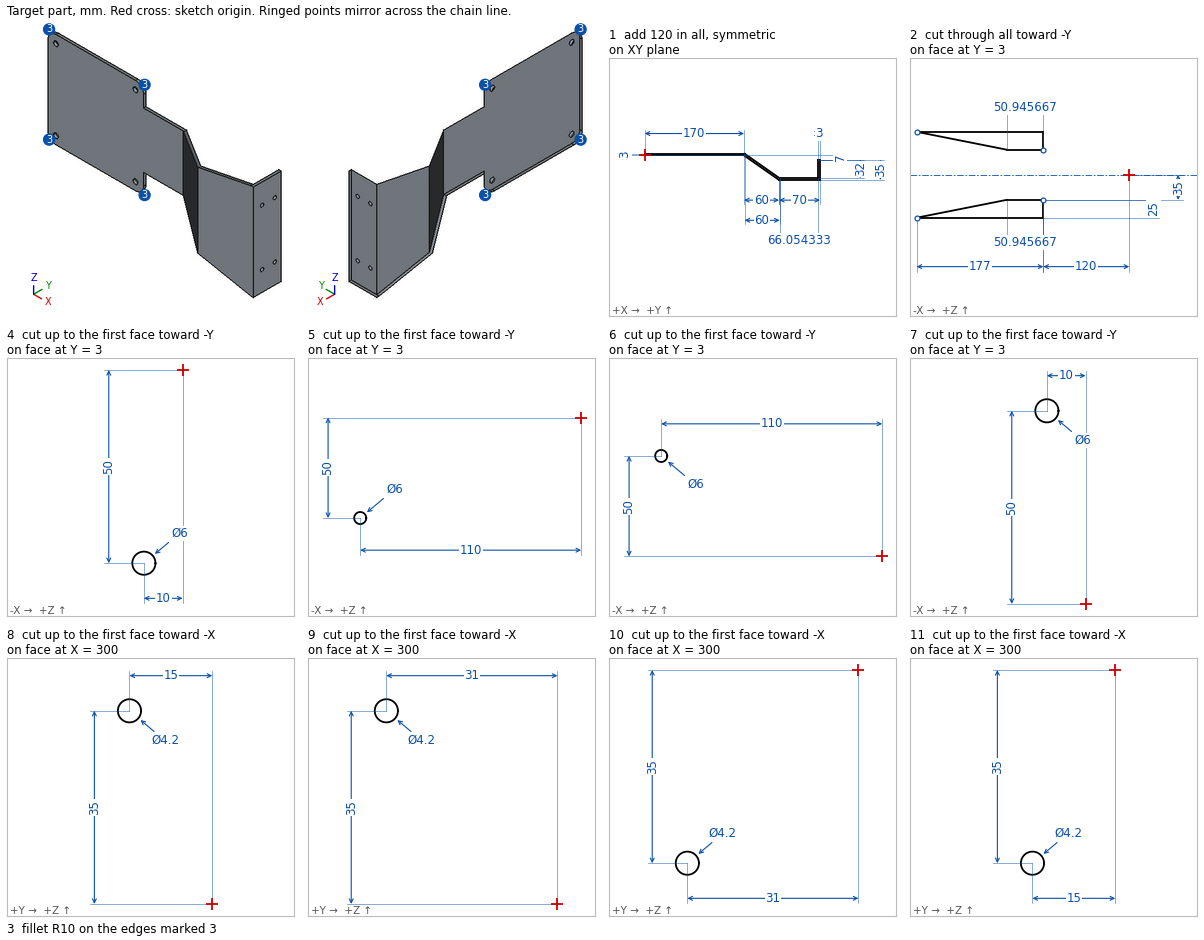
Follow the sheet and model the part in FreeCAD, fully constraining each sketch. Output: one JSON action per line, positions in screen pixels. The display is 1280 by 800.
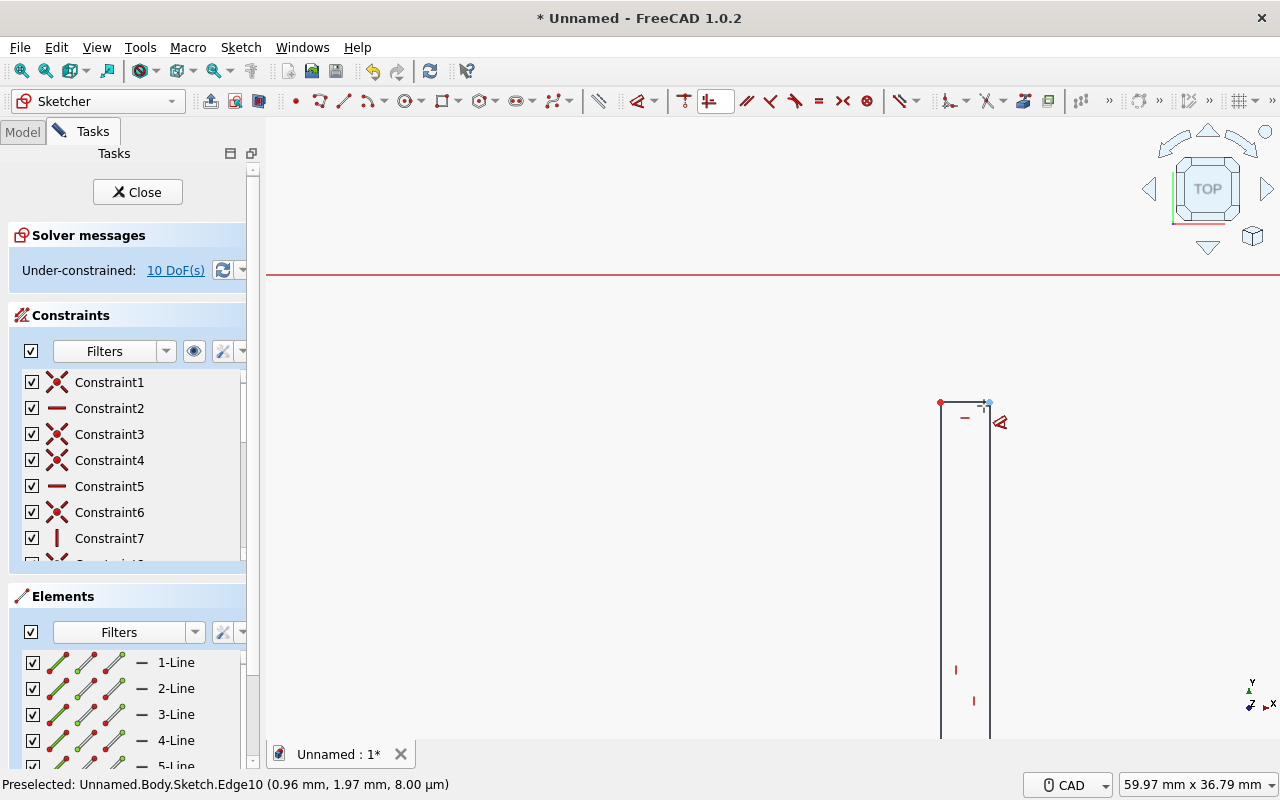
{"action": "left_click", "coordinate": [975, 402]}
{"action": "left_click", "coordinate": [965, 368]}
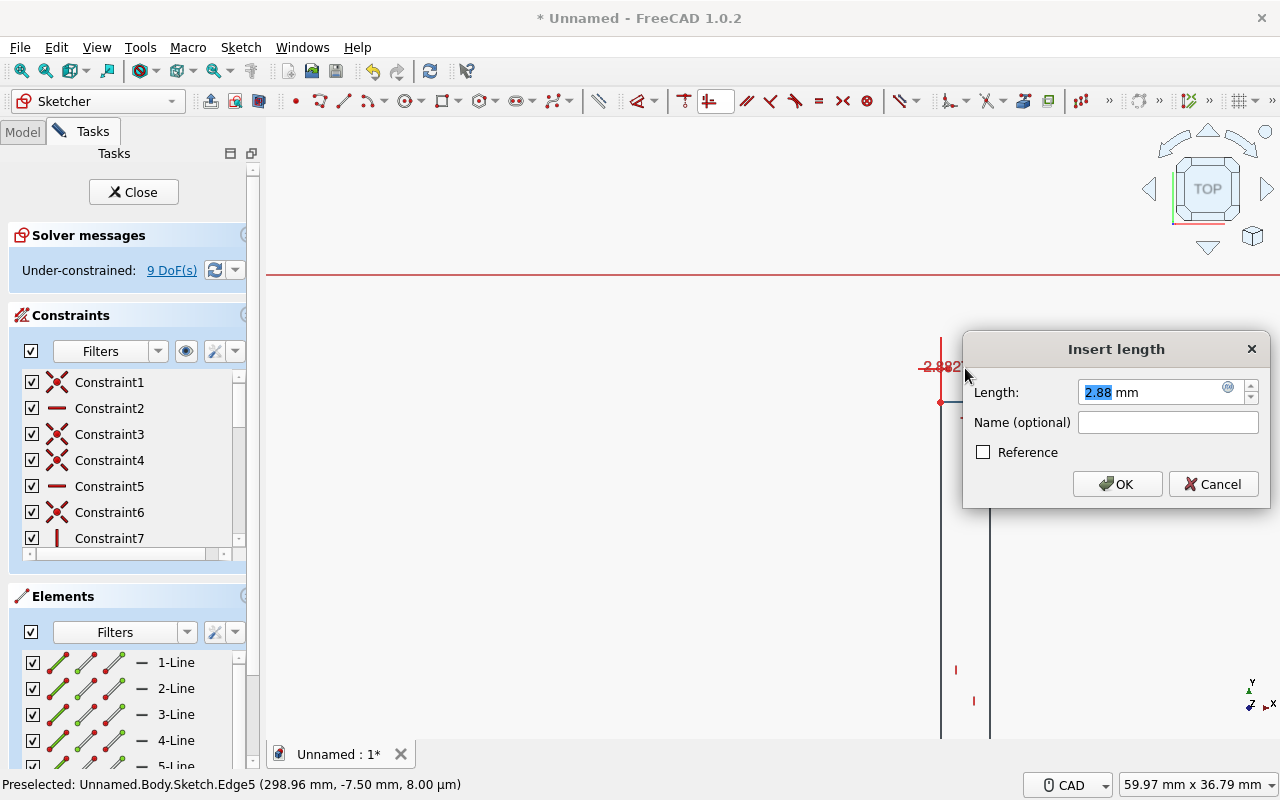
{"action": "type", "text": "3"}
{"action": "key", "text": "Return"}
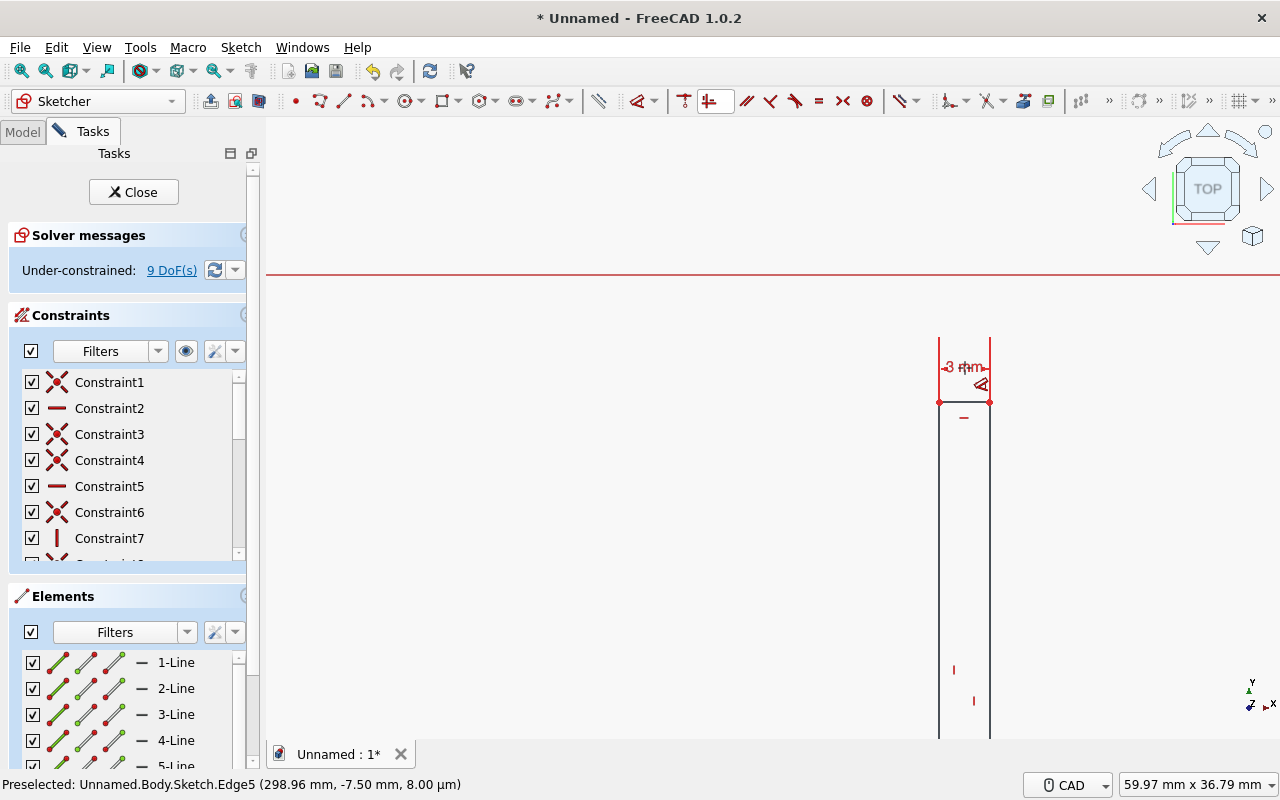
{"action": "scroll", "coordinate": [985, 406], "scroll_direction": "down", "scroll_amount": 11}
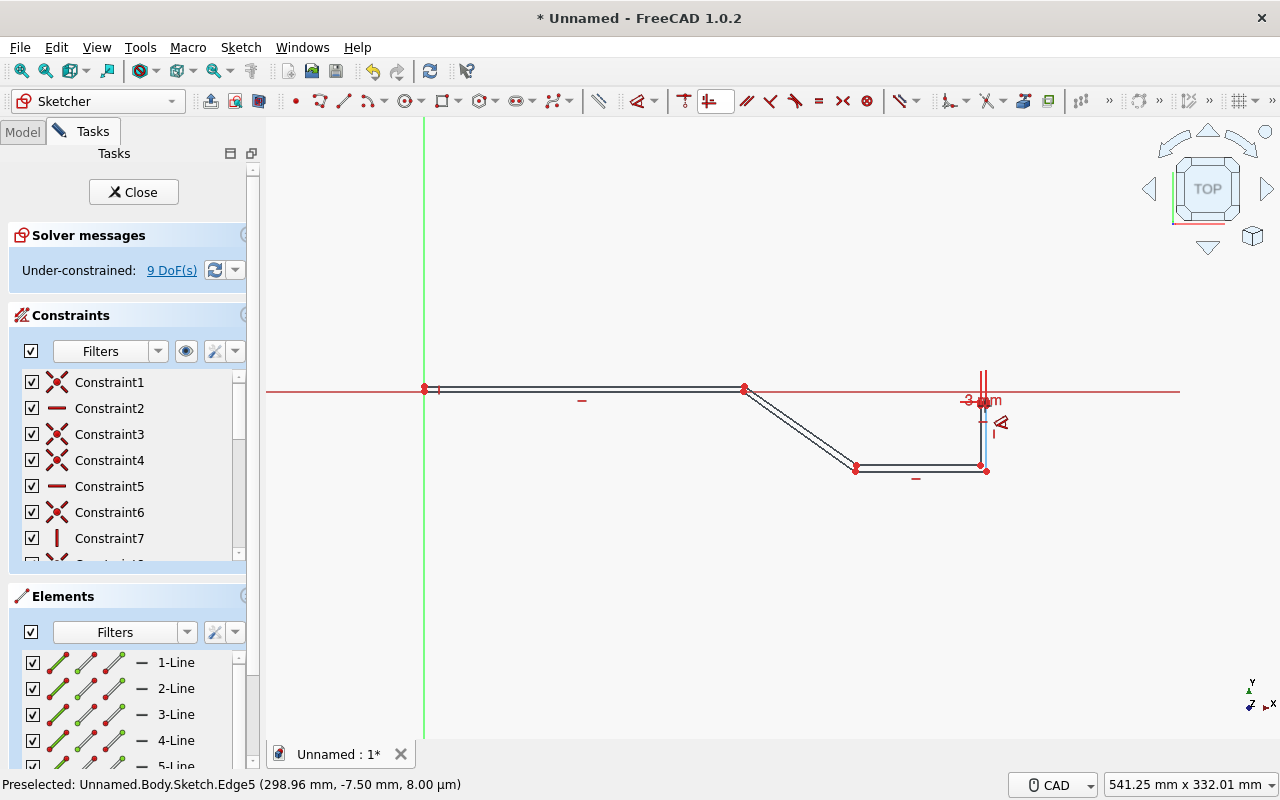
{"action": "scroll", "coordinate": [424, 388], "scroll_direction": "up", "scroll_amount": 11}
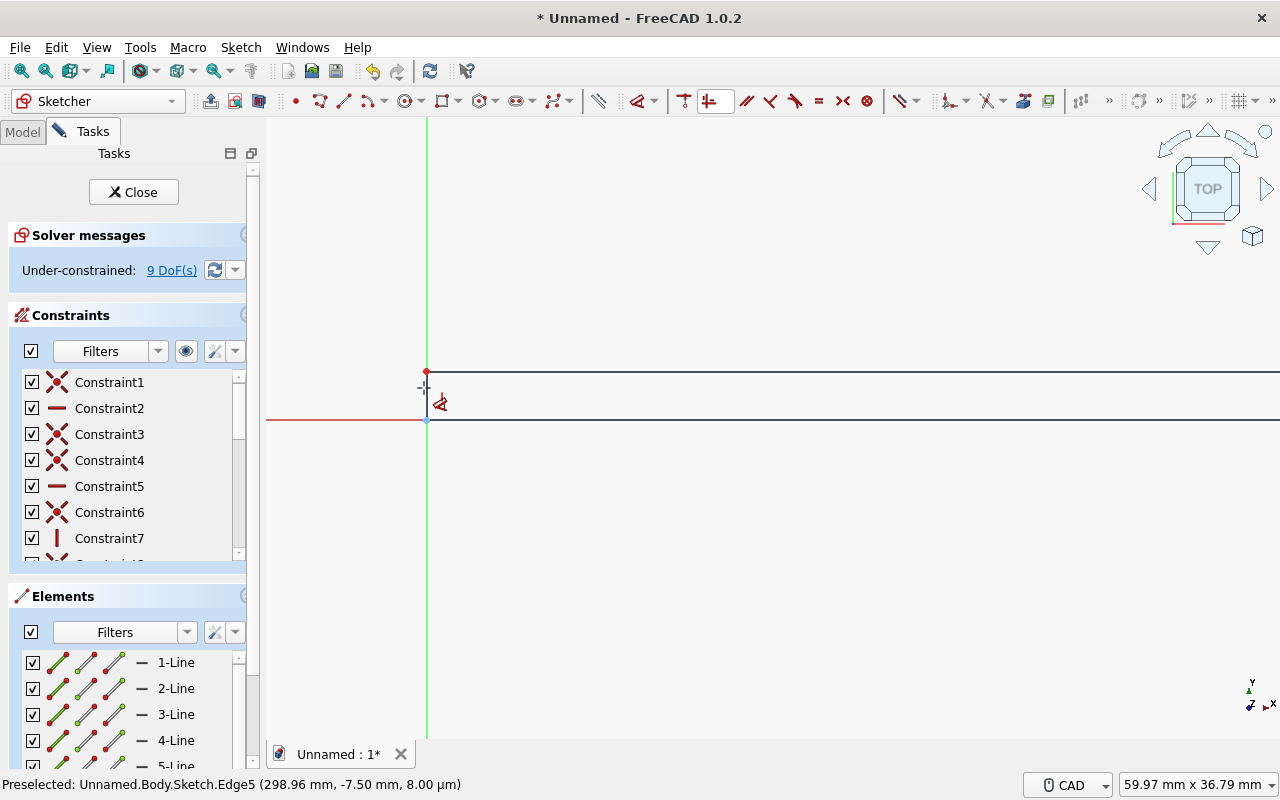
{"action": "left_click", "coordinate": [427, 386]}
{"action": "left_click", "coordinate": [393, 396]}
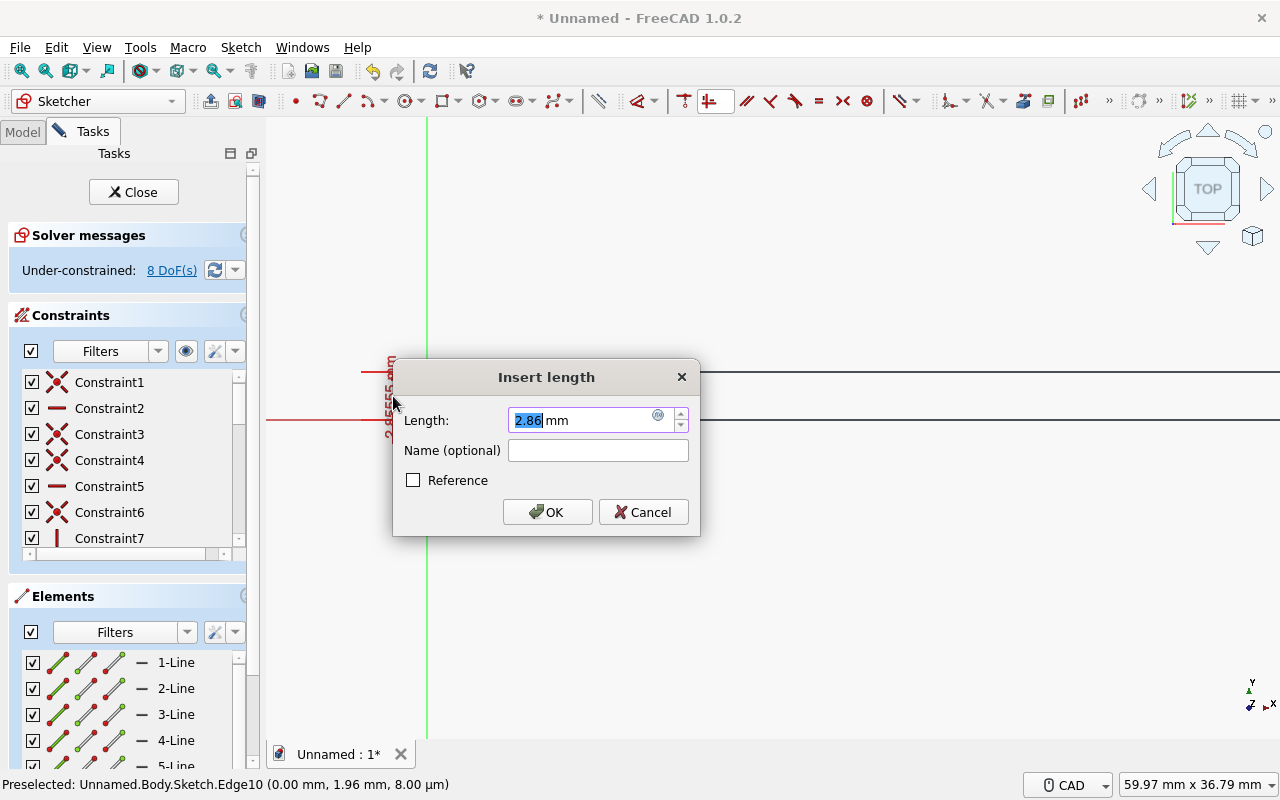
{"action": "type", "text": "3"}
{"action": "key", "text": "Return"}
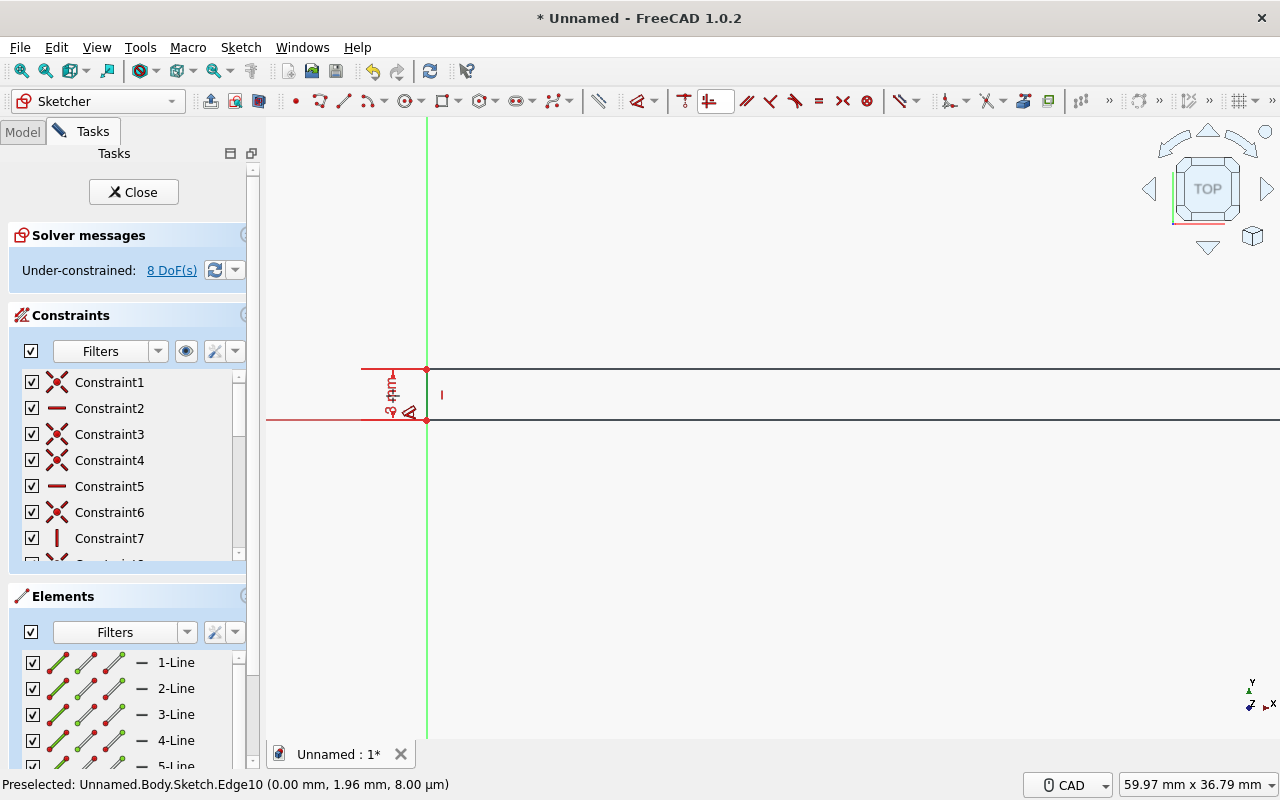
{"action": "scroll", "coordinate": [423, 388], "scroll_direction": "down", "scroll_amount": 11}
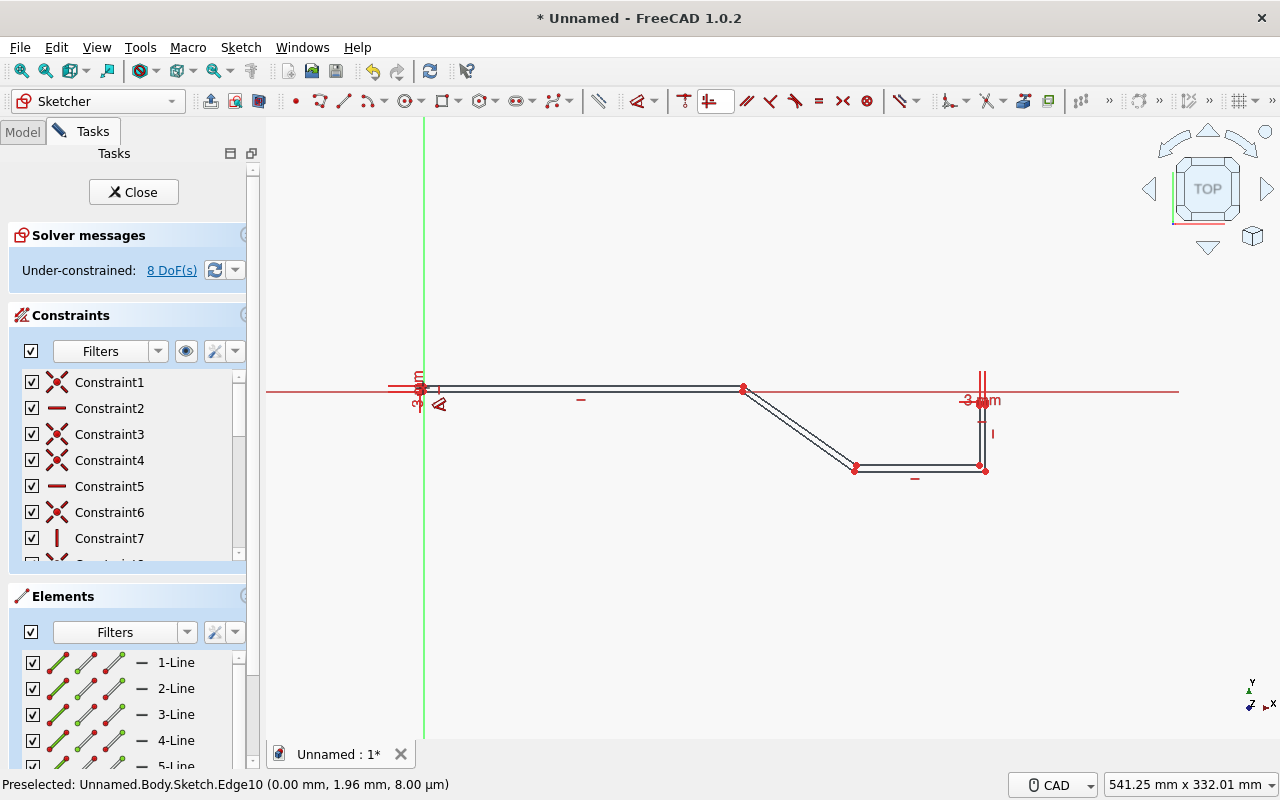
{"action": "scroll", "coordinate": [894, 472], "scroll_direction": "up", "scroll_amount": 4}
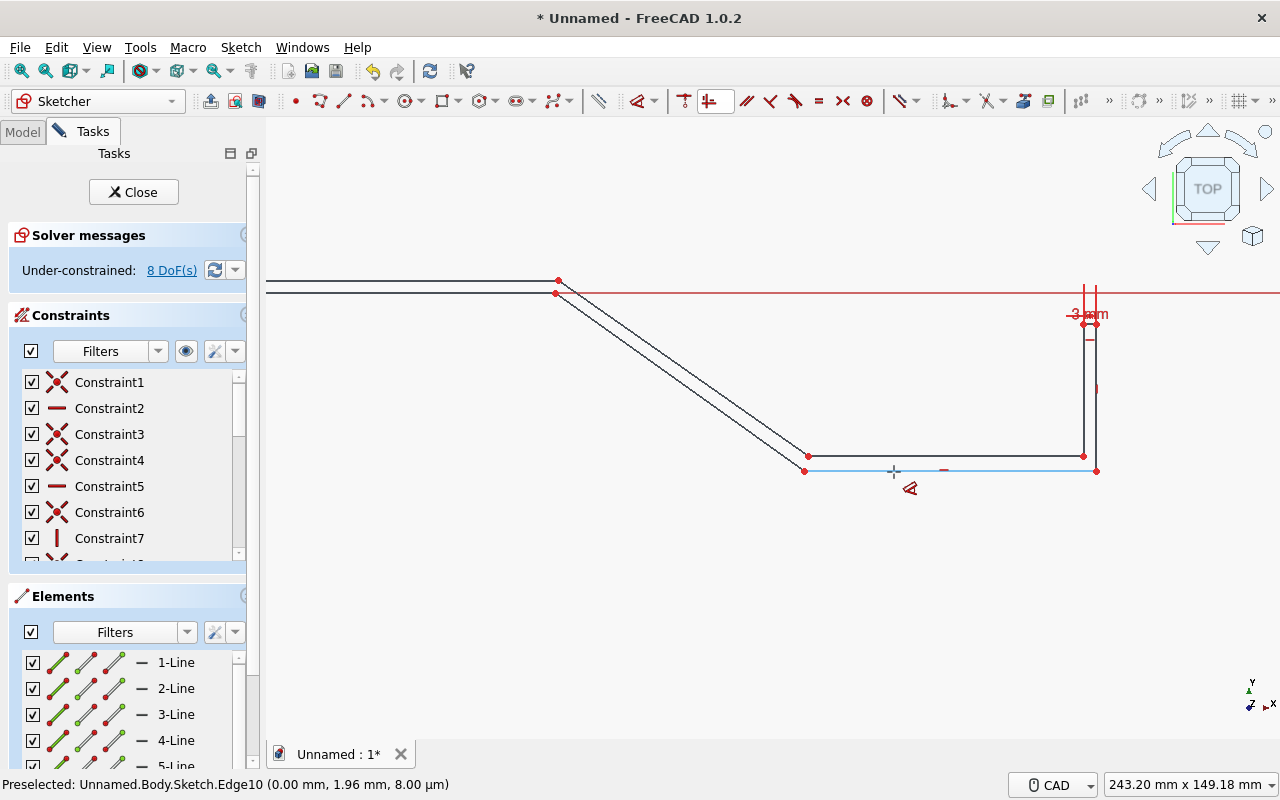
{"action": "left_click", "coordinate": [892, 471]}
{"action": "left_click", "coordinate": [951, 505]}